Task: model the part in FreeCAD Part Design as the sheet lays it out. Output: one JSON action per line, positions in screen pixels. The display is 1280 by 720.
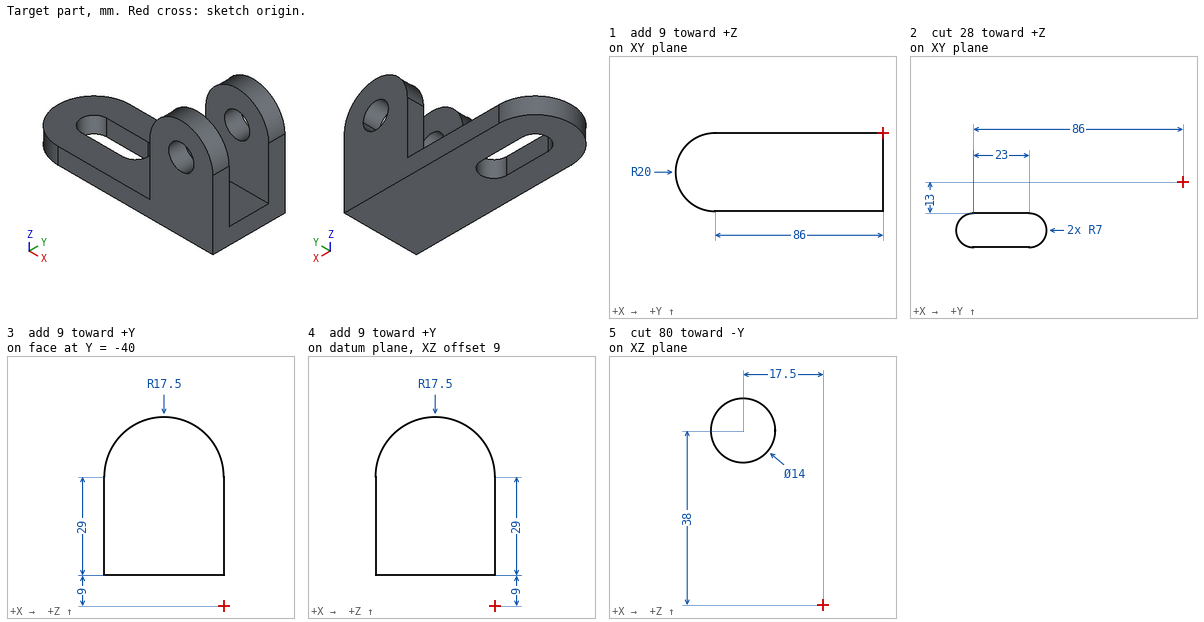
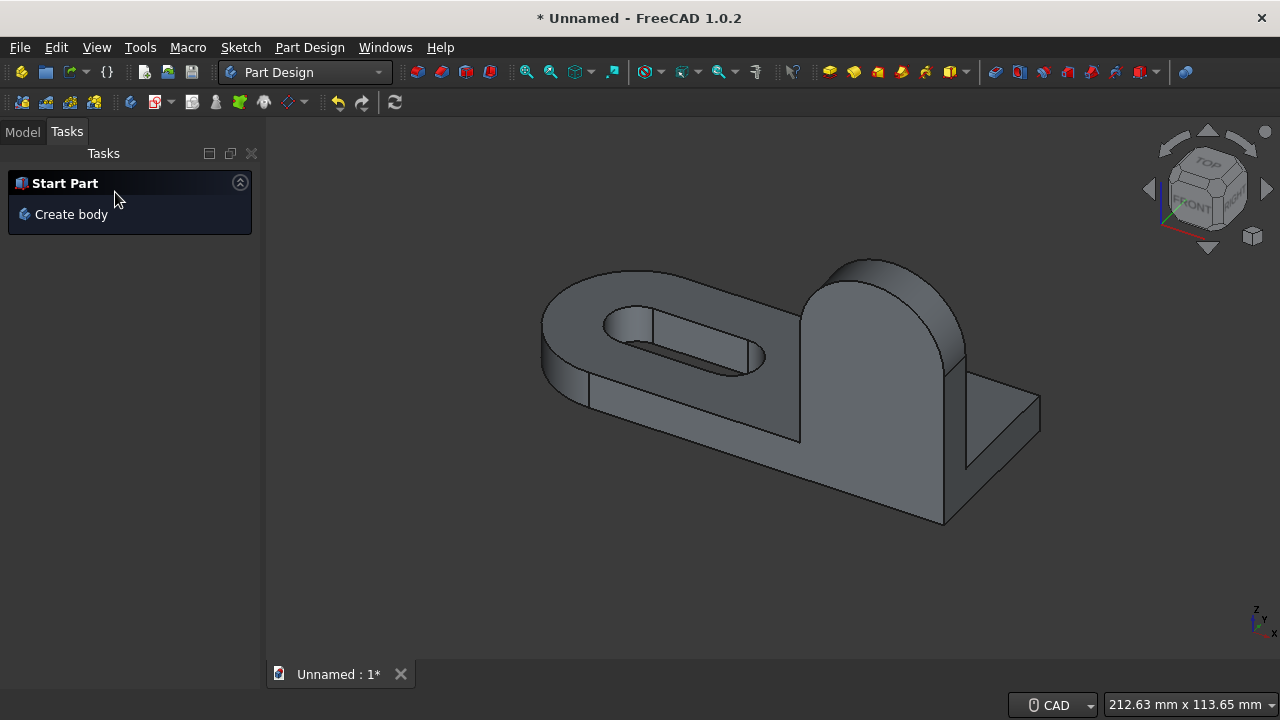
{"action": "left_click", "coordinate": [528, 72]}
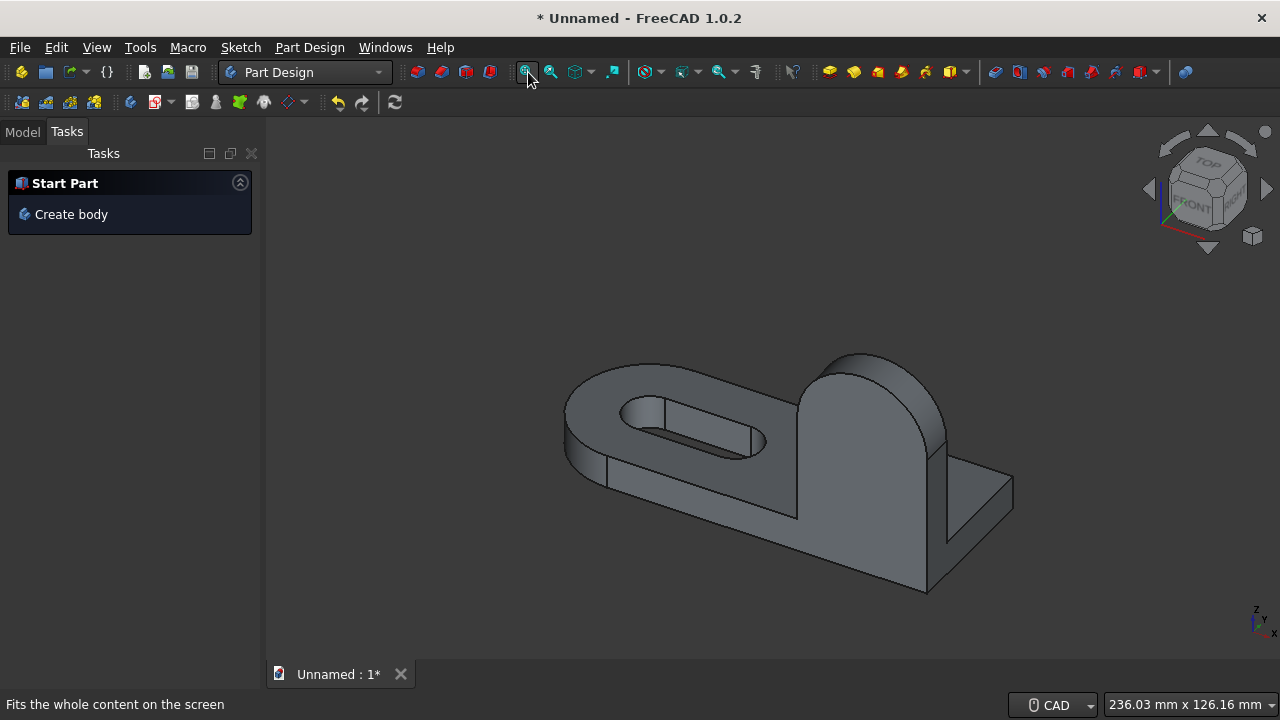
{"action": "left_click", "coordinate": [23, 131]}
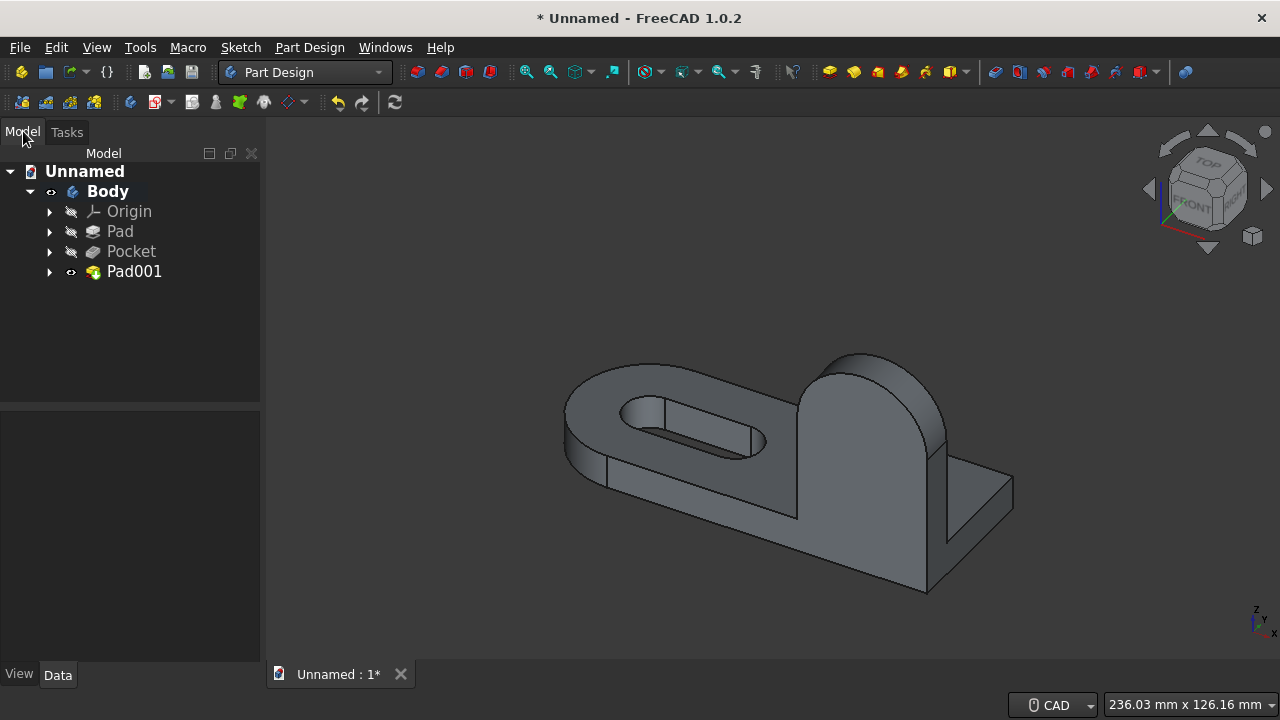
{"action": "left_click", "coordinate": [50, 212]}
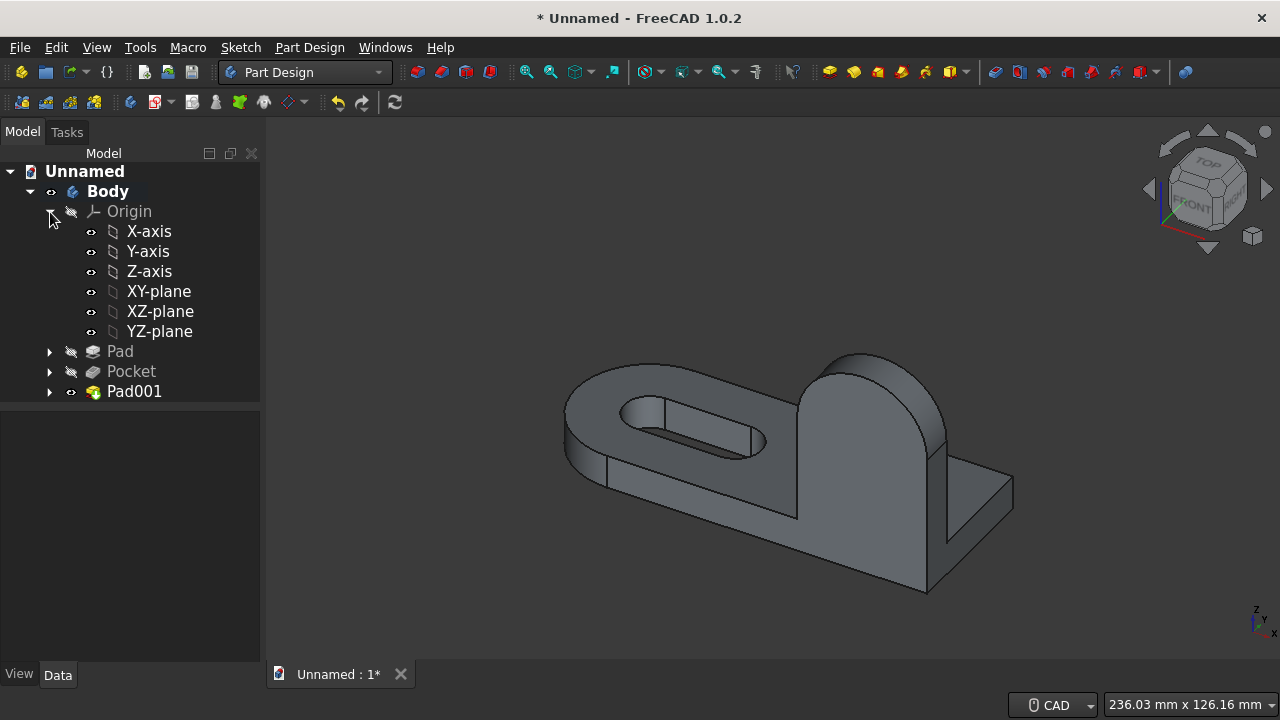
{"action": "left_click", "coordinate": [136, 312]}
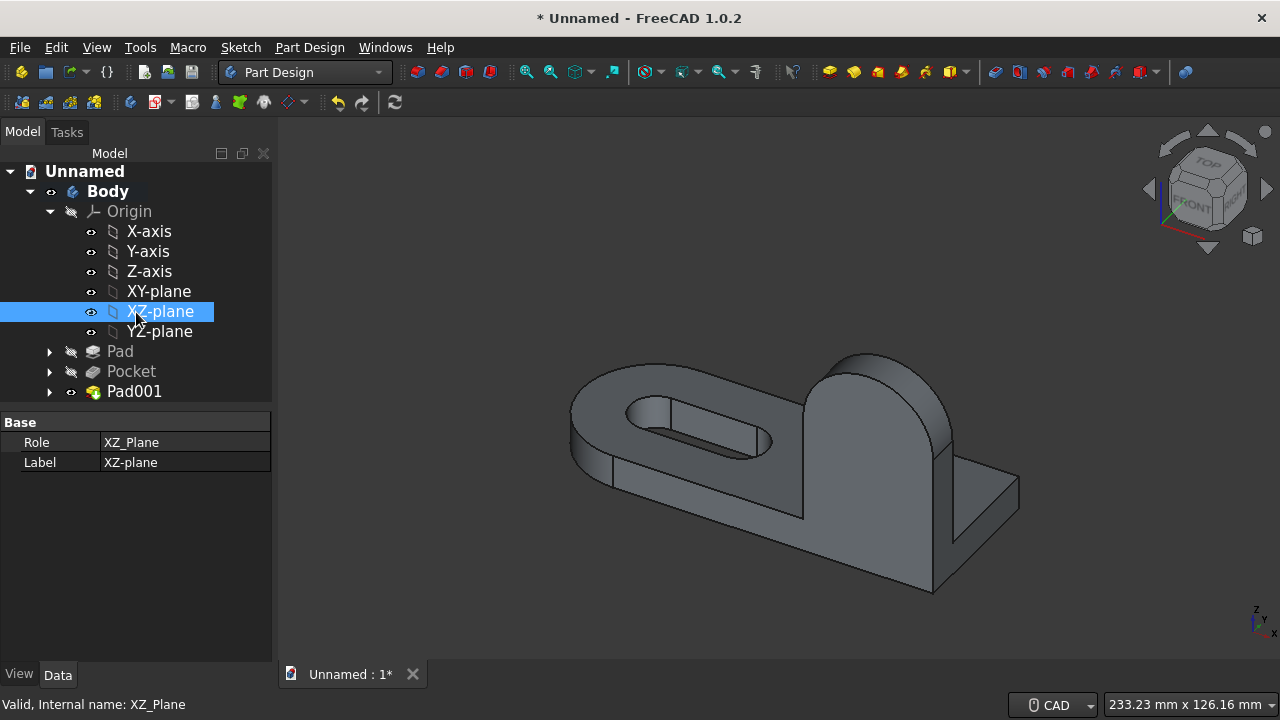
{"action": "left_click", "coordinate": [288, 102]}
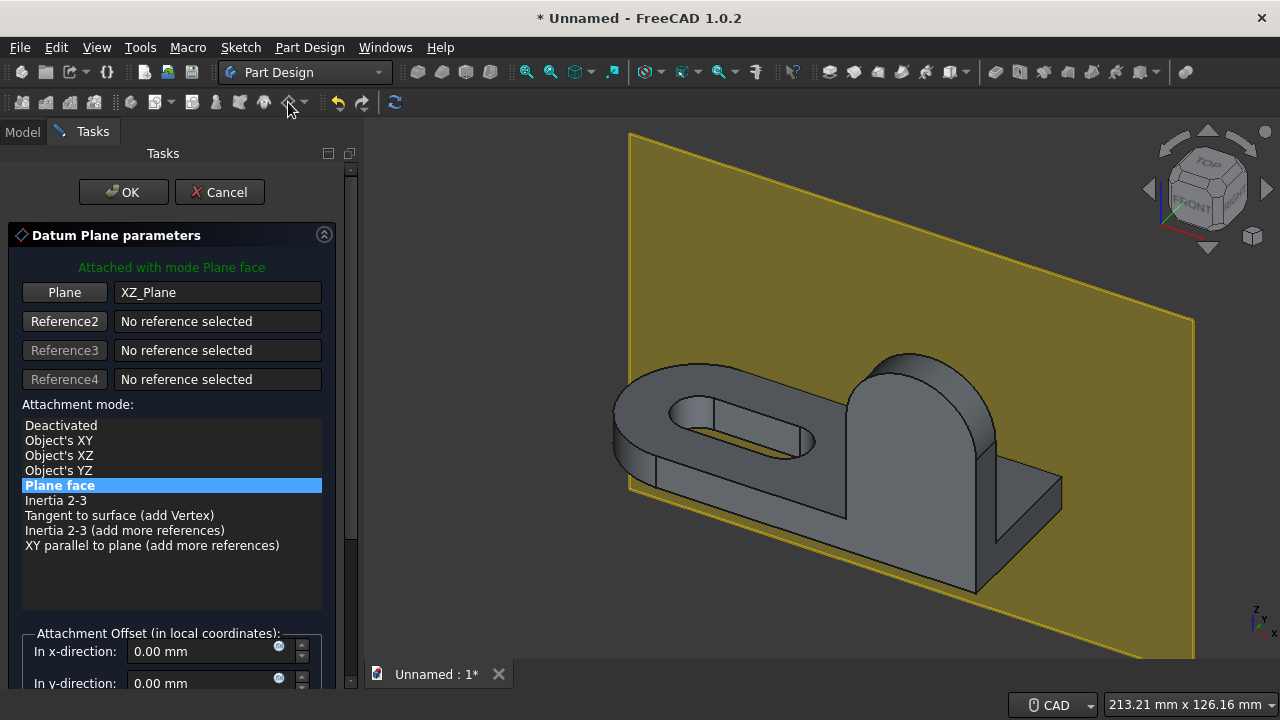
{"action": "scroll", "coordinate": [351, 426], "scroll_direction": "down", "scroll_amount": 2}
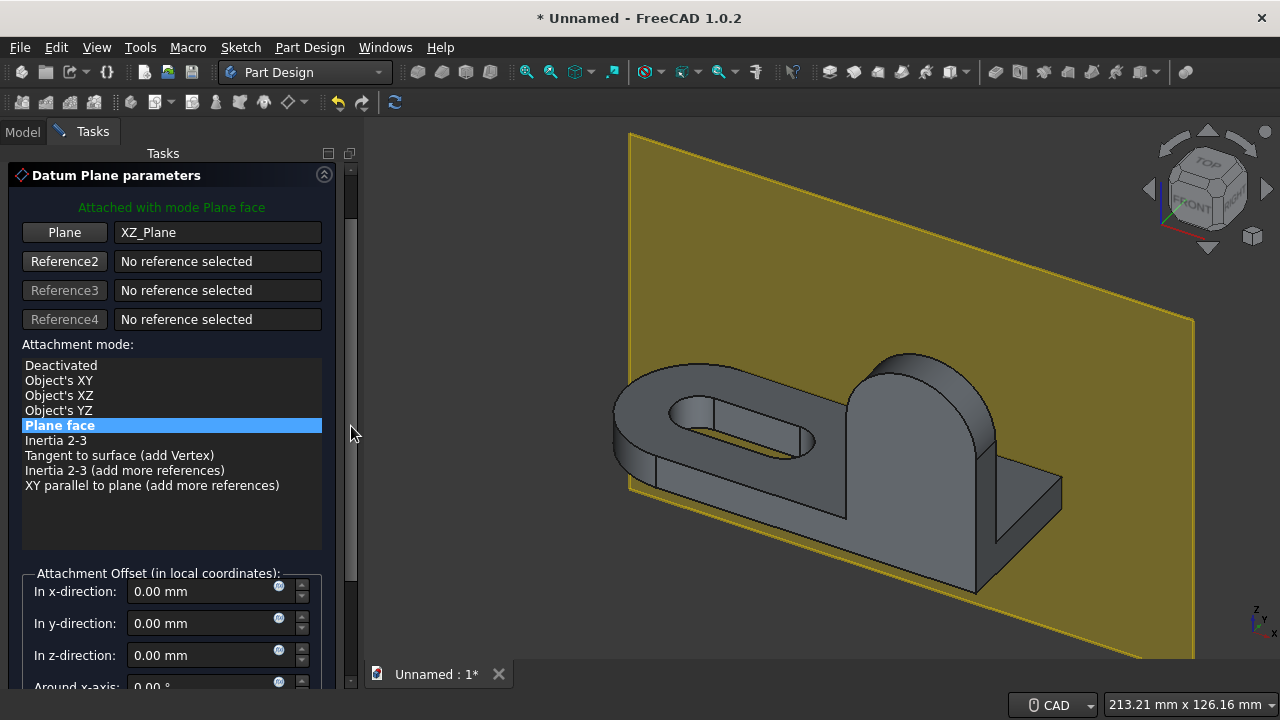
{"action": "triple_click", "coordinate": [210, 595]}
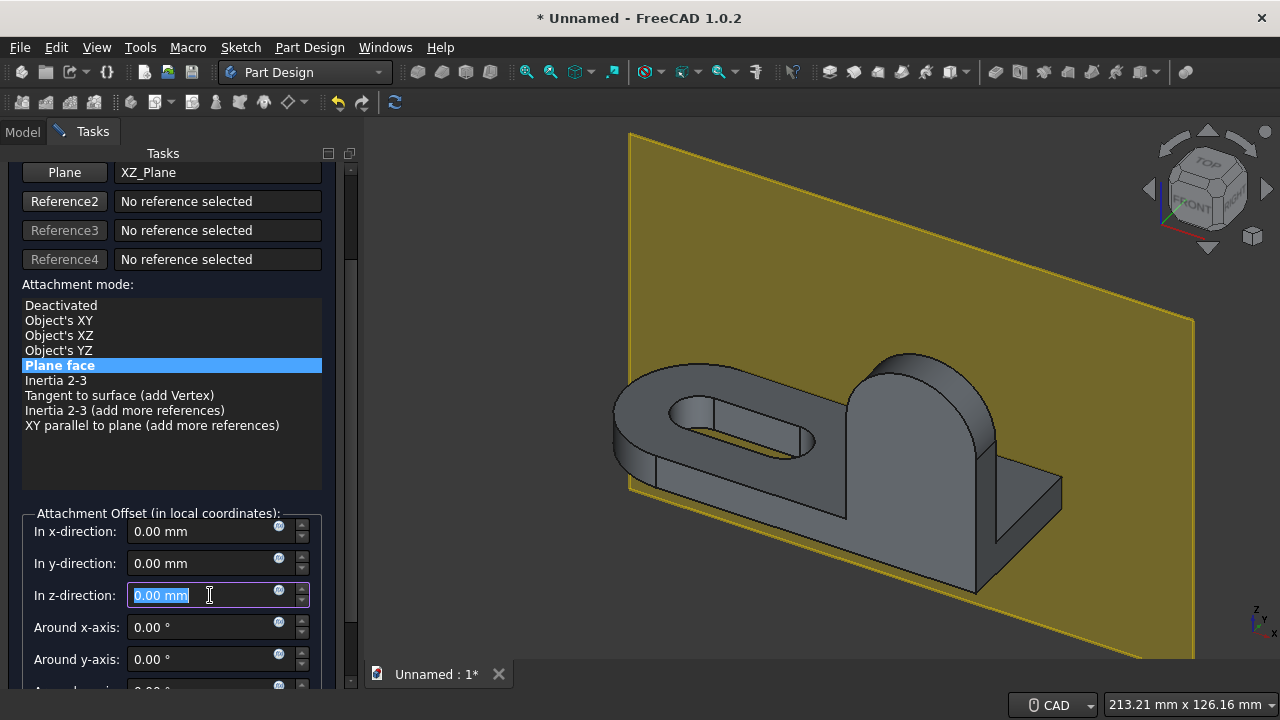
{"action": "type", "text": "9"}
{"action": "key", "text": "Tab"}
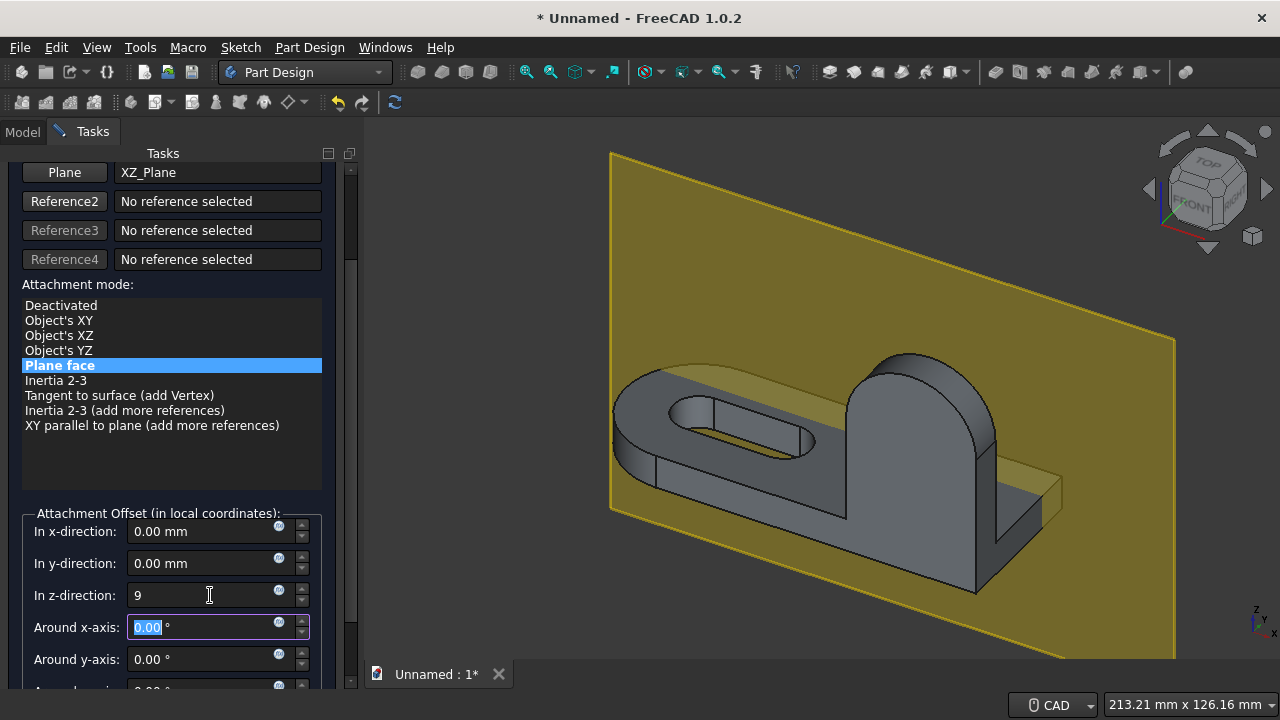
{"action": "scroll", "coordinate": [351, 426], "scroll_direction": "up", "scroll_amount": 3}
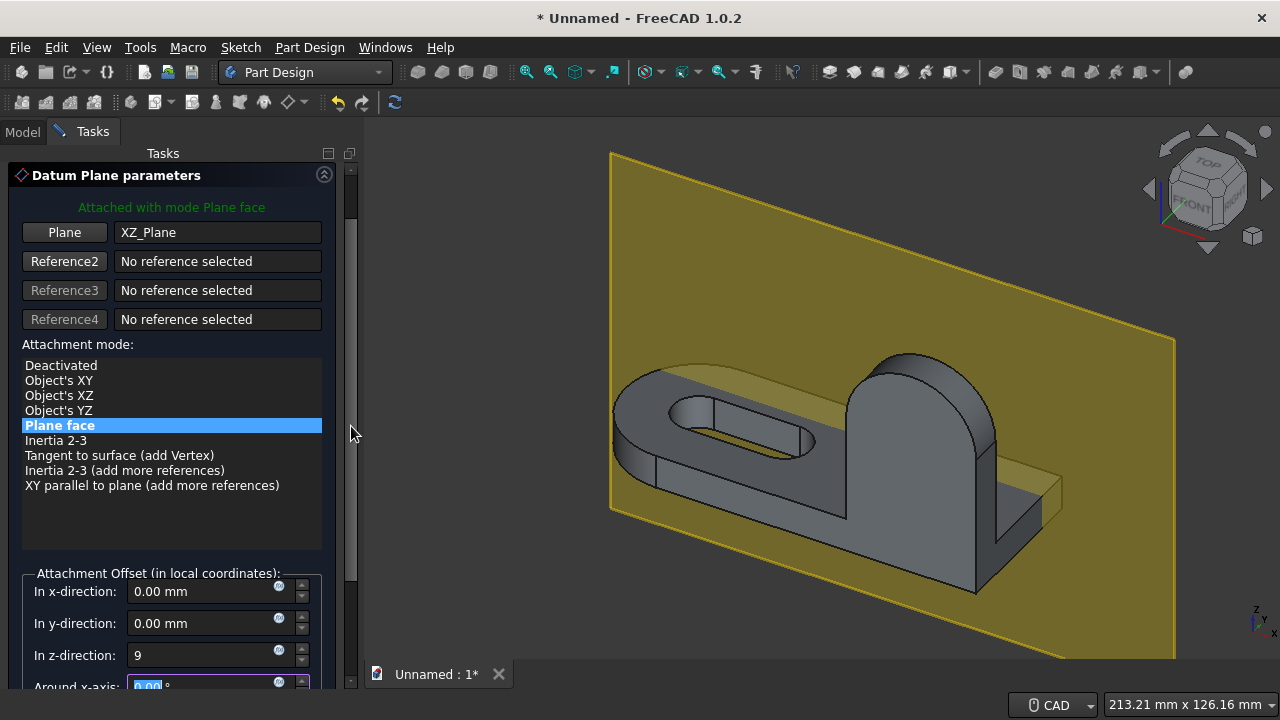
{"action": "left_click", "coordinate": [124, 192]}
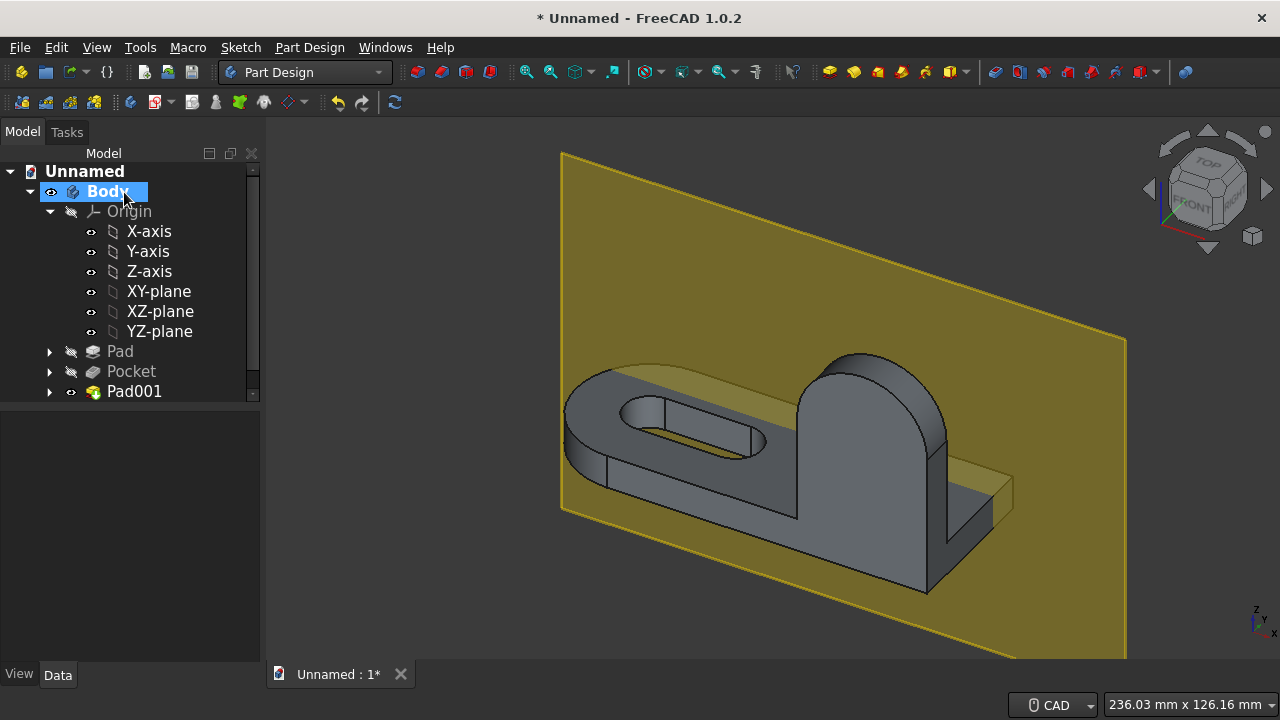
{"action": "scroll", "coordinate": [100, 287], "scroll_direction": "down", "scroll_amount": 3}